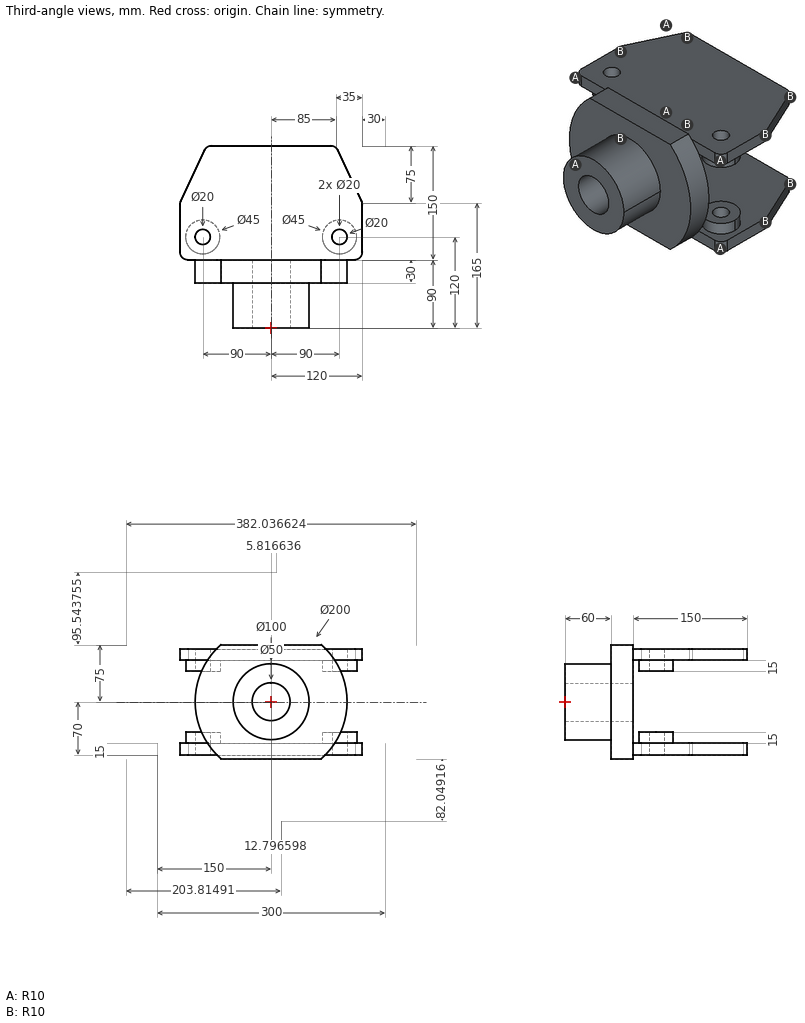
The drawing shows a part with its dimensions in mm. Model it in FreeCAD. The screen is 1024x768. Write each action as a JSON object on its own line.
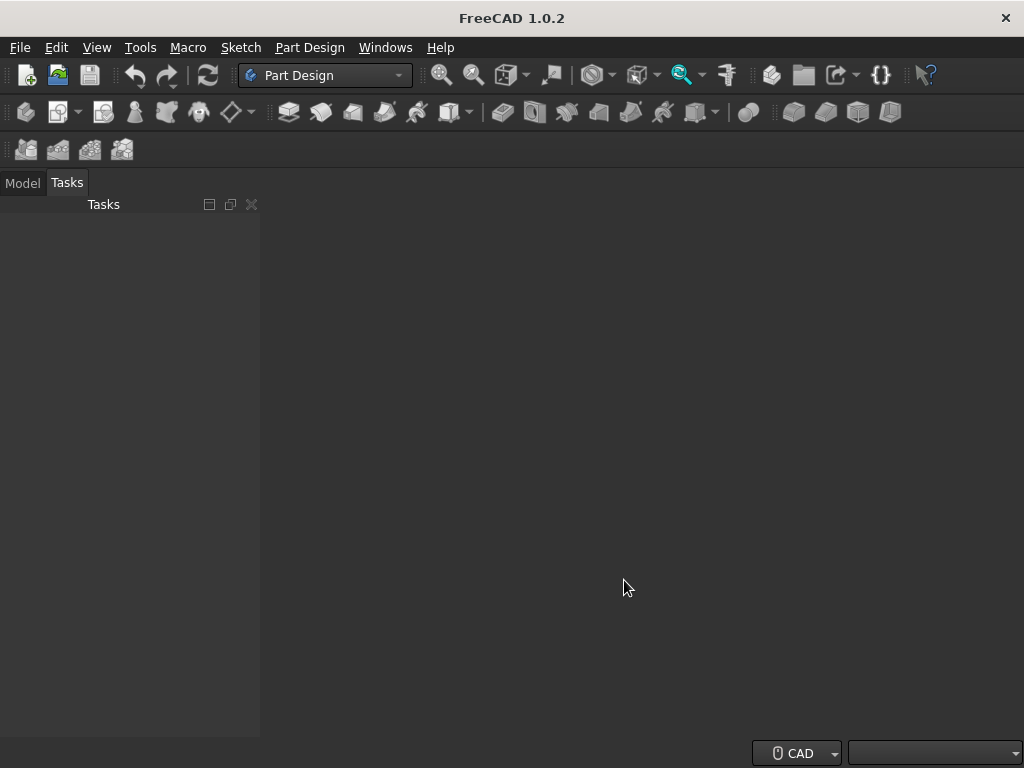
{"action": "left_click", "coordinate": [26, 76]}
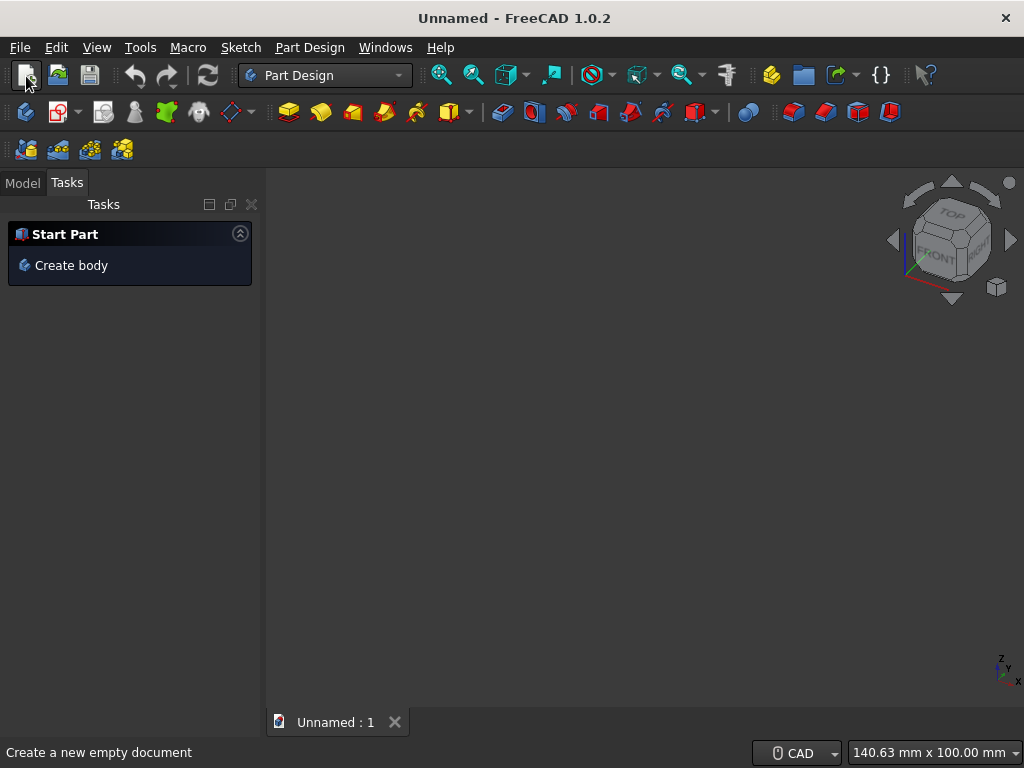
{"action": "left_click", "coordinate": [58, 112]}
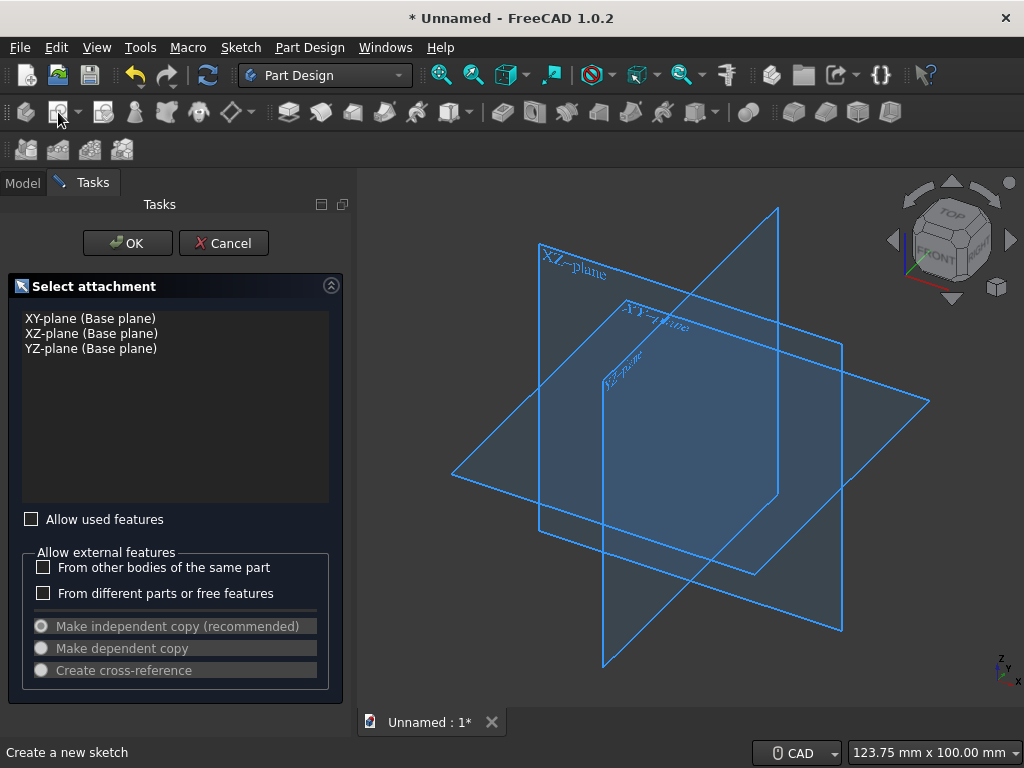
{"action": "left_click", "coordinate": [82, 334]}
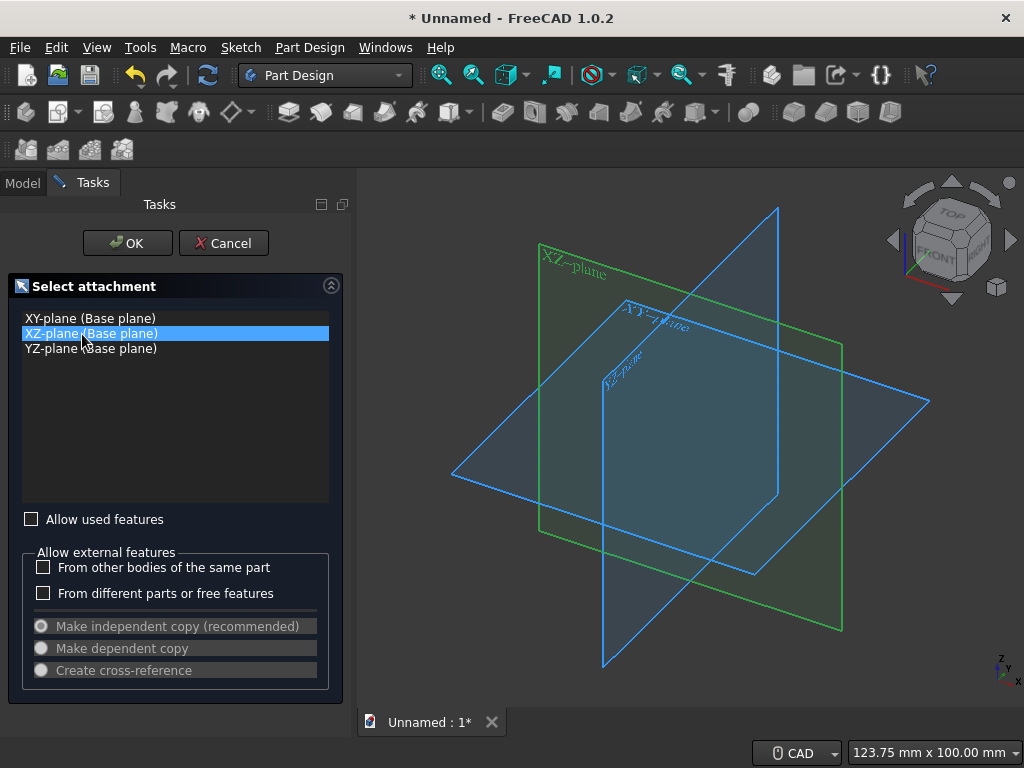
{"action": "left_click", "coordinate": [128, 243]}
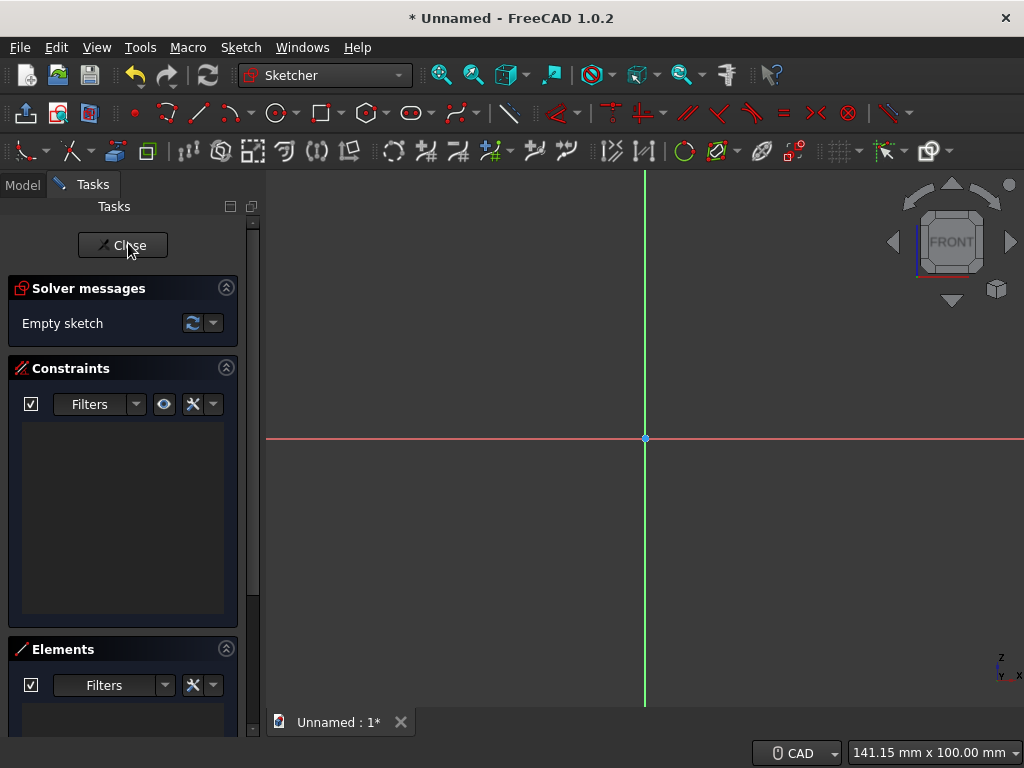
{"action": "scroll", "coordinate": [437, 438], "scroll_direction": "down", "scroll_amount": 2}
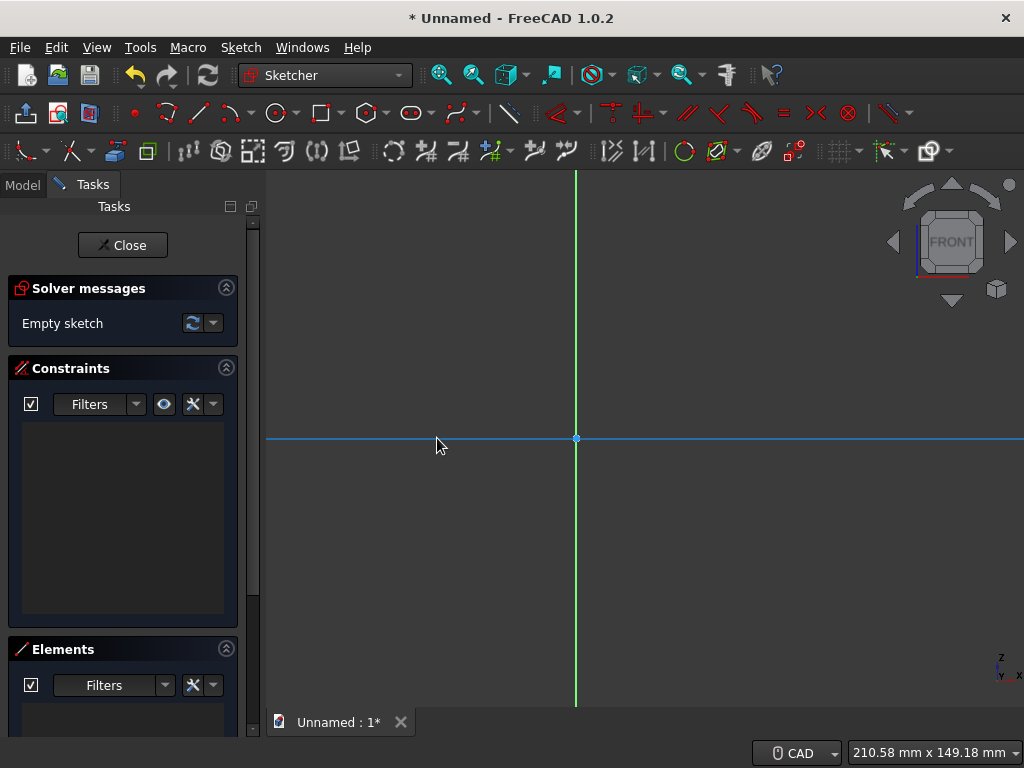
{"action": "left_click", "coordinate": [276, 114]}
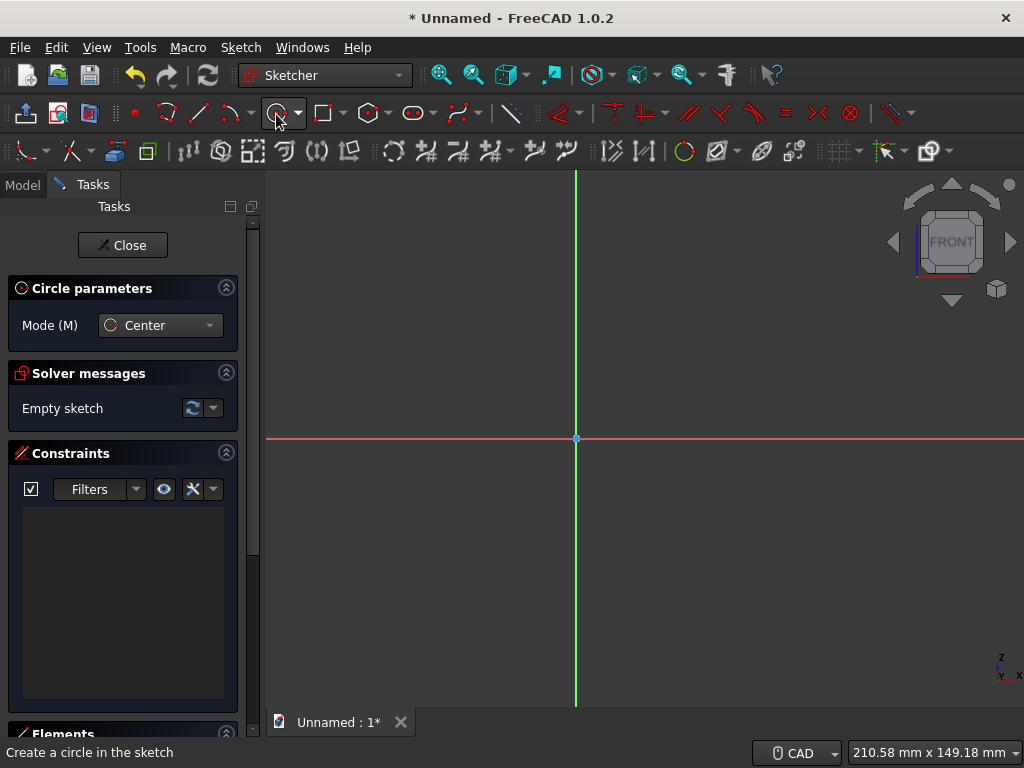
{"action": "left_click", "coordinate": [577, 438]}
{"action": "left_click", "coordinate": [704, 311]}
{"action": "key", "text": "Escape"}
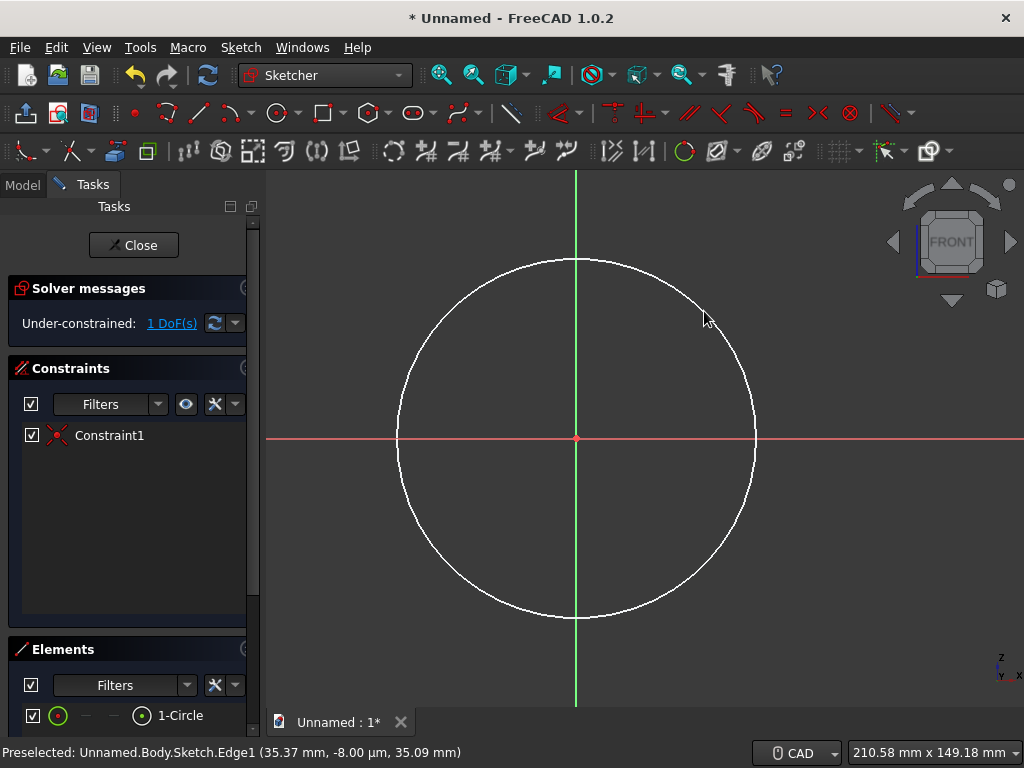
{"action": "key", "text": "d"}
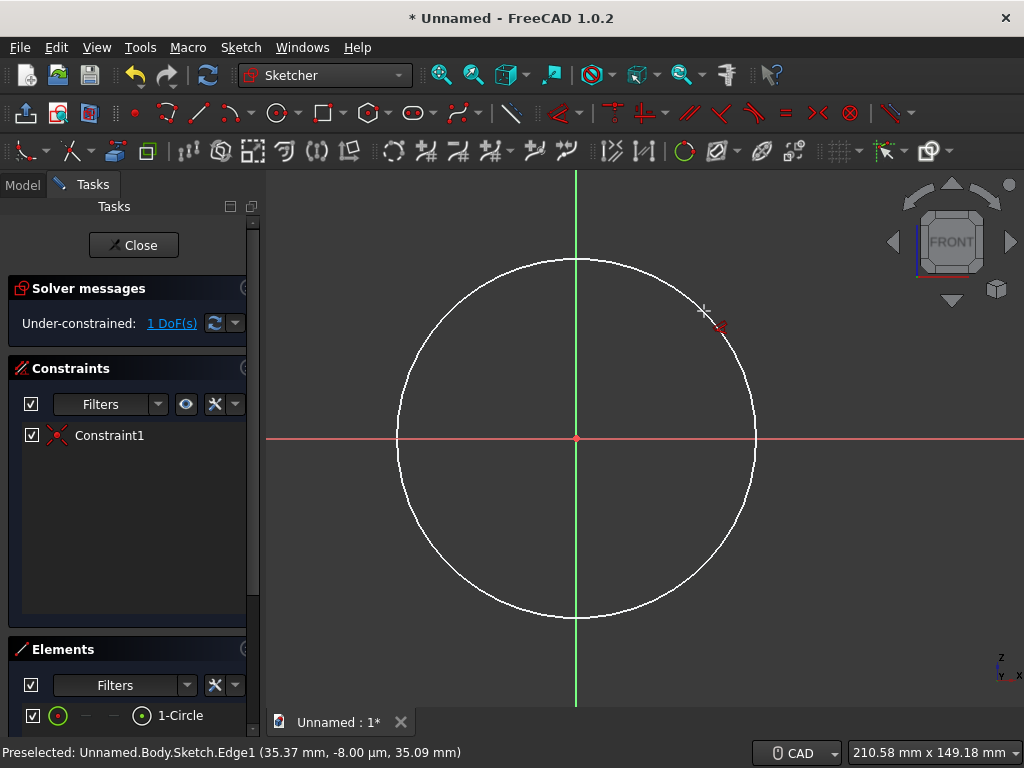
{"action": "left_click", "coordinate": [703, 311]}
{"action": "left_click", "coordinate": [726, 288]}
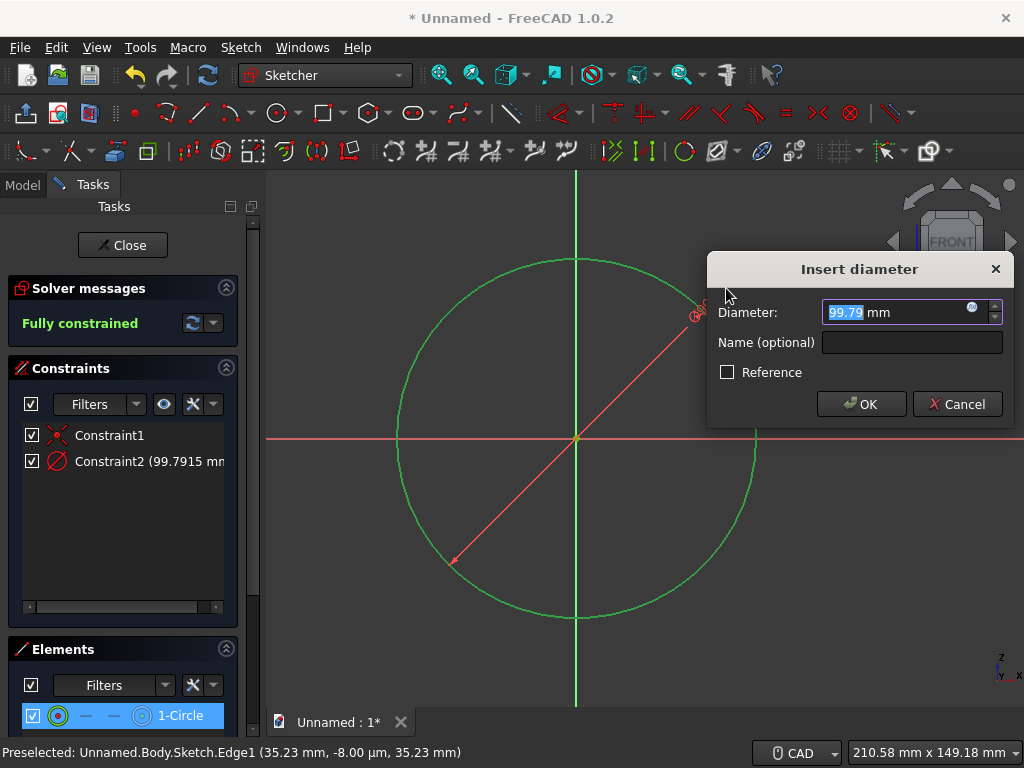
{"action": "type", "text": "100"}
{"action": "key", "text": "Return"}
{"action": "key", "text": "Escape"}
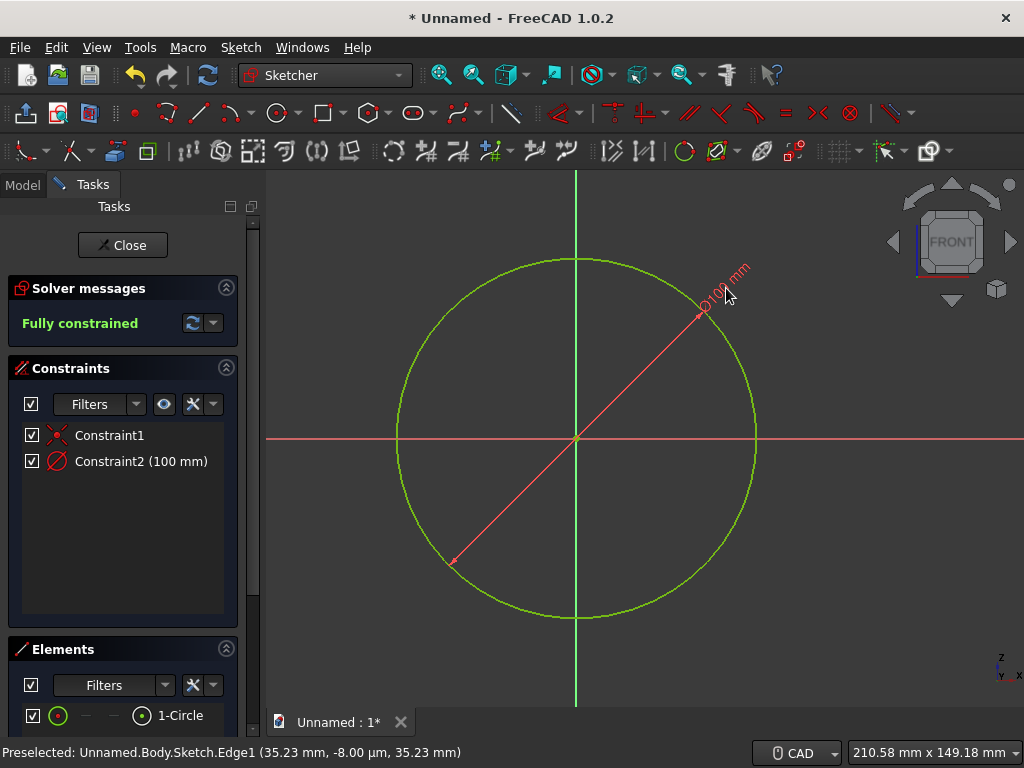
{"action": "left_click", "coordinate": [123, 245]}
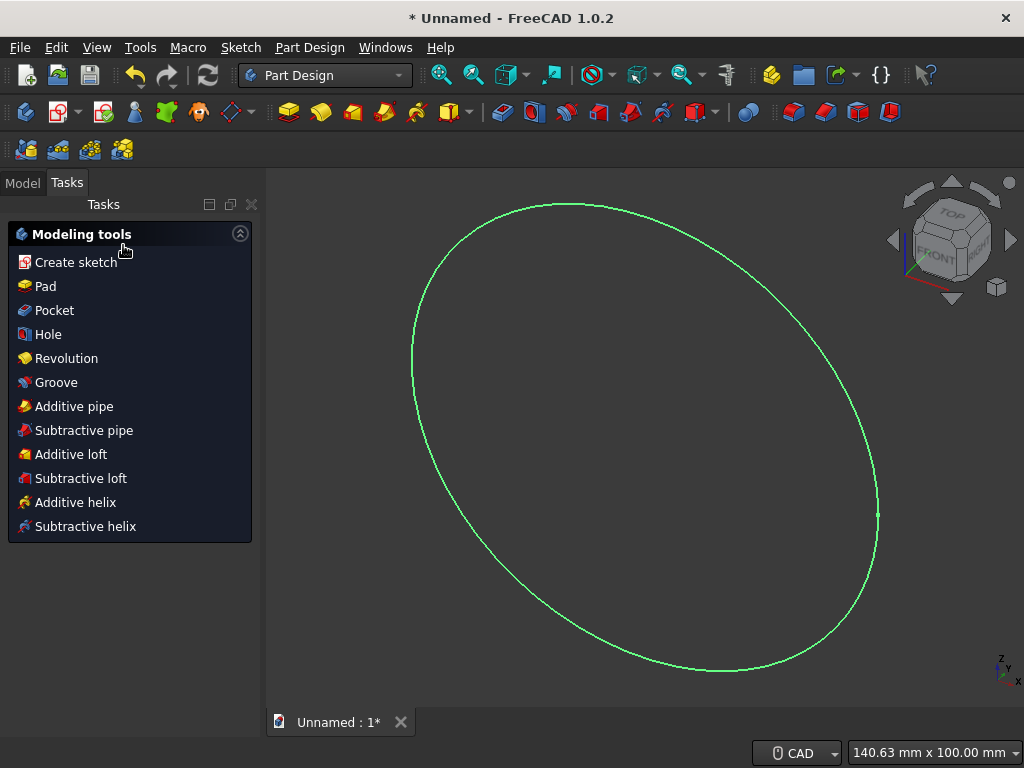
{"action": "left_click", "coordinate": [290, 112]}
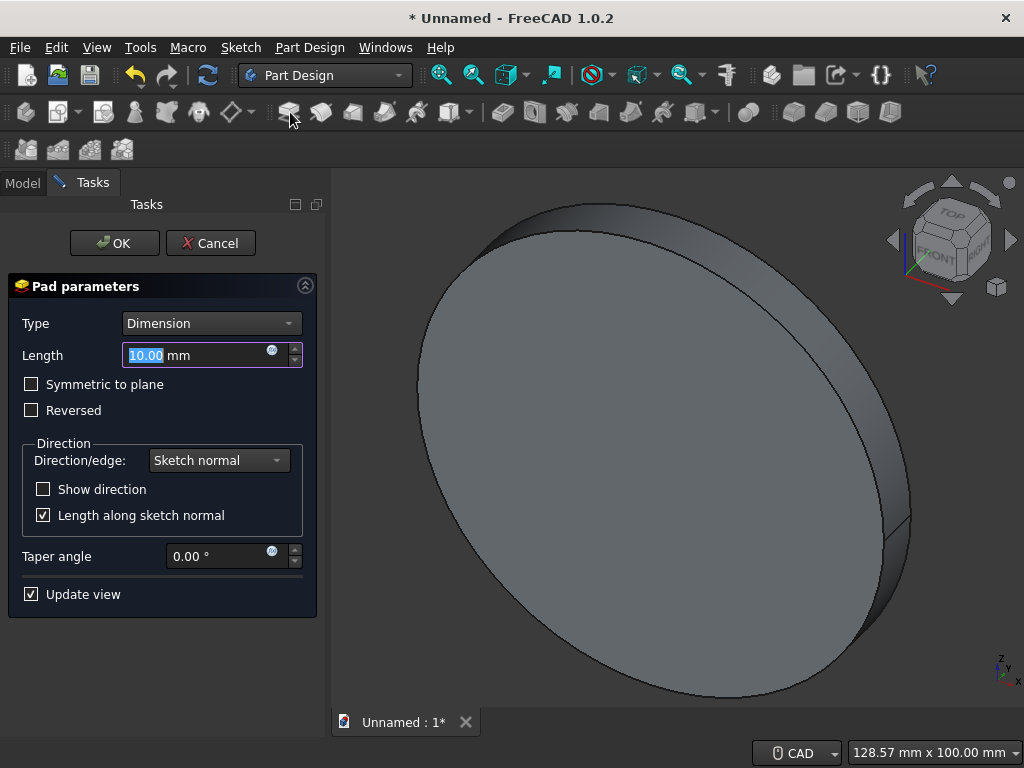
{"action": "type", "text": "60"}
{"action": "key", "text": "Tab"}